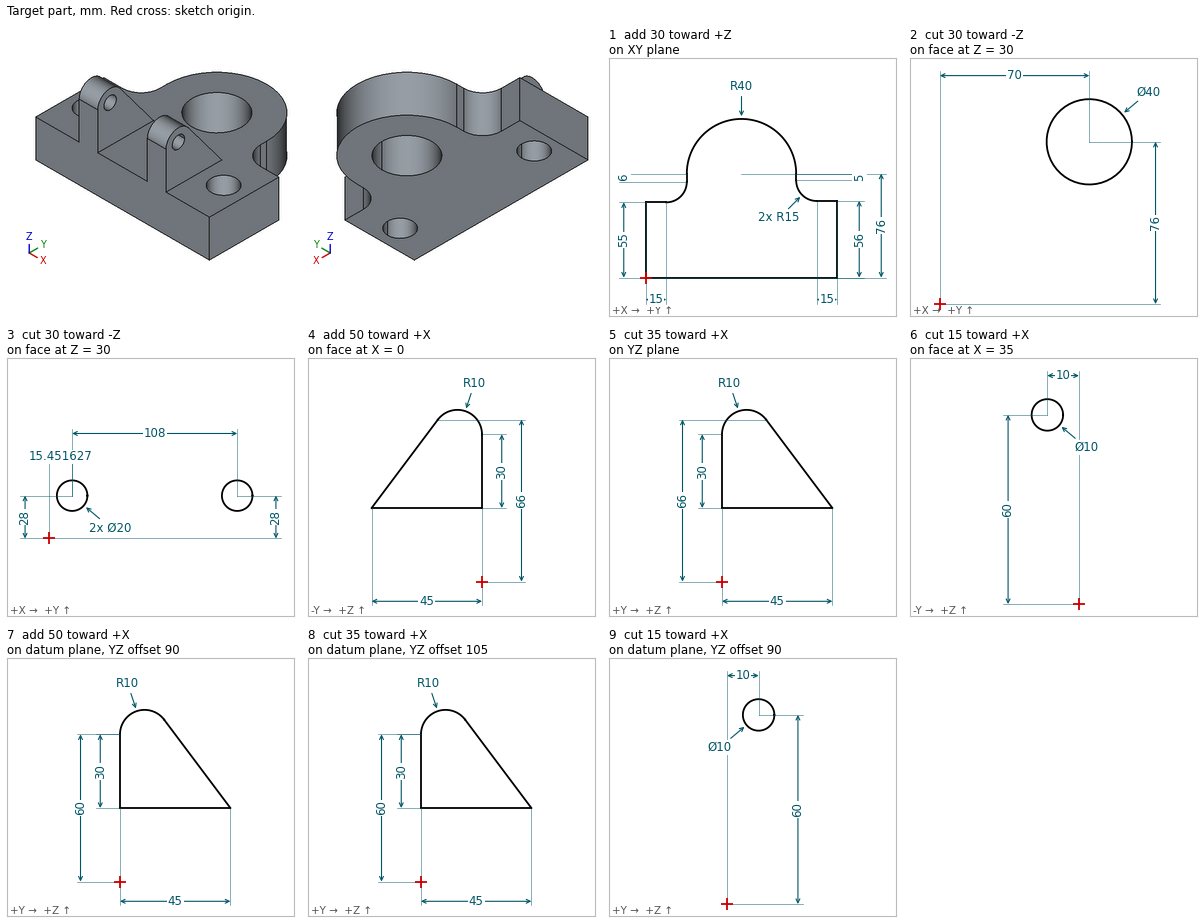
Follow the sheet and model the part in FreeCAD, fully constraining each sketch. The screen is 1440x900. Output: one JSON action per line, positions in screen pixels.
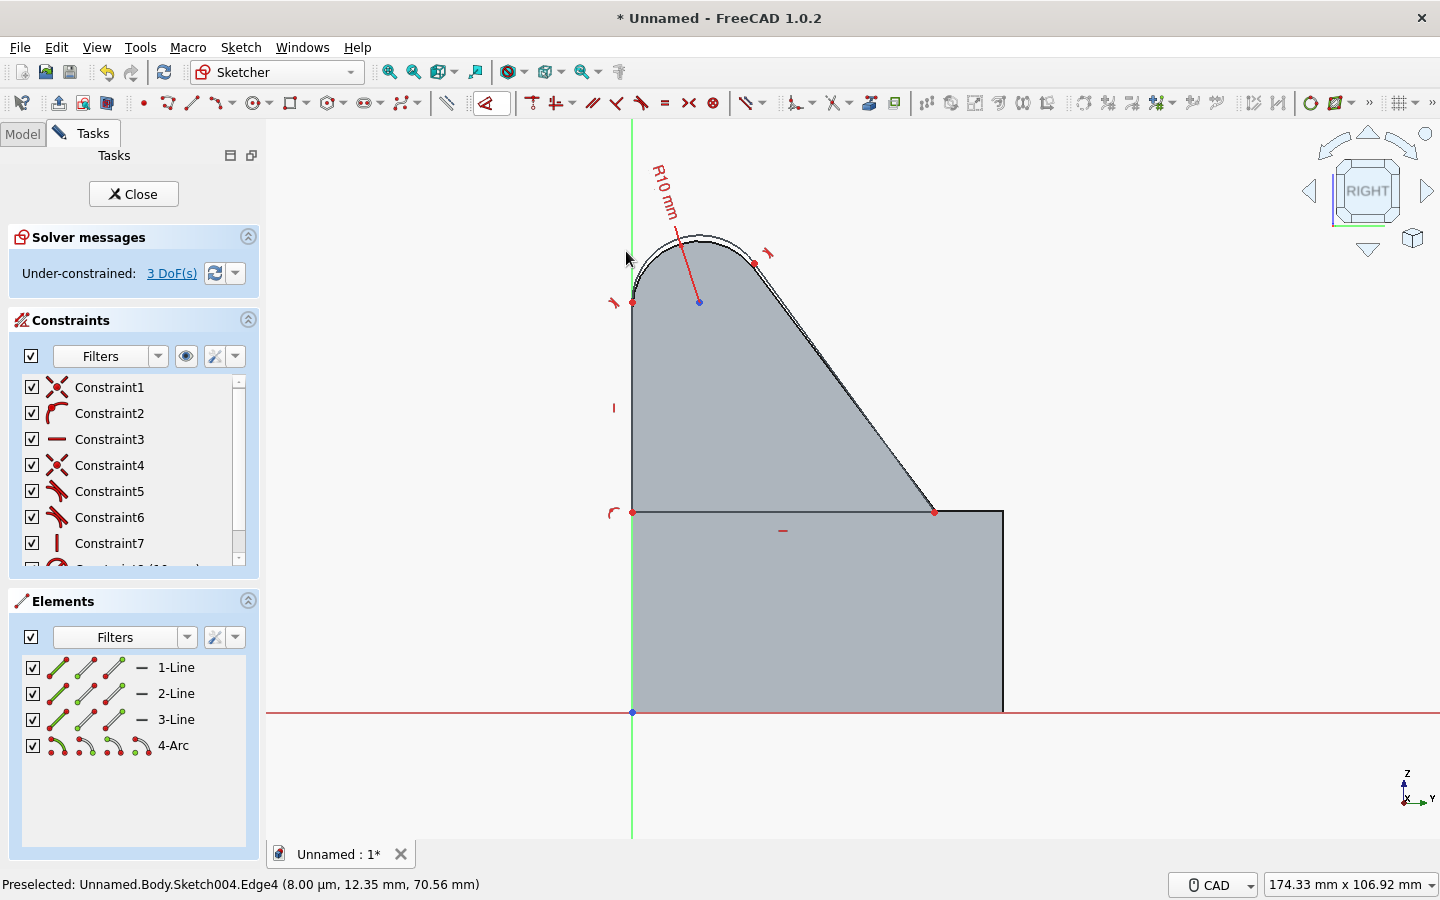
{"action": "left_click", "coordinate": [844, 512]}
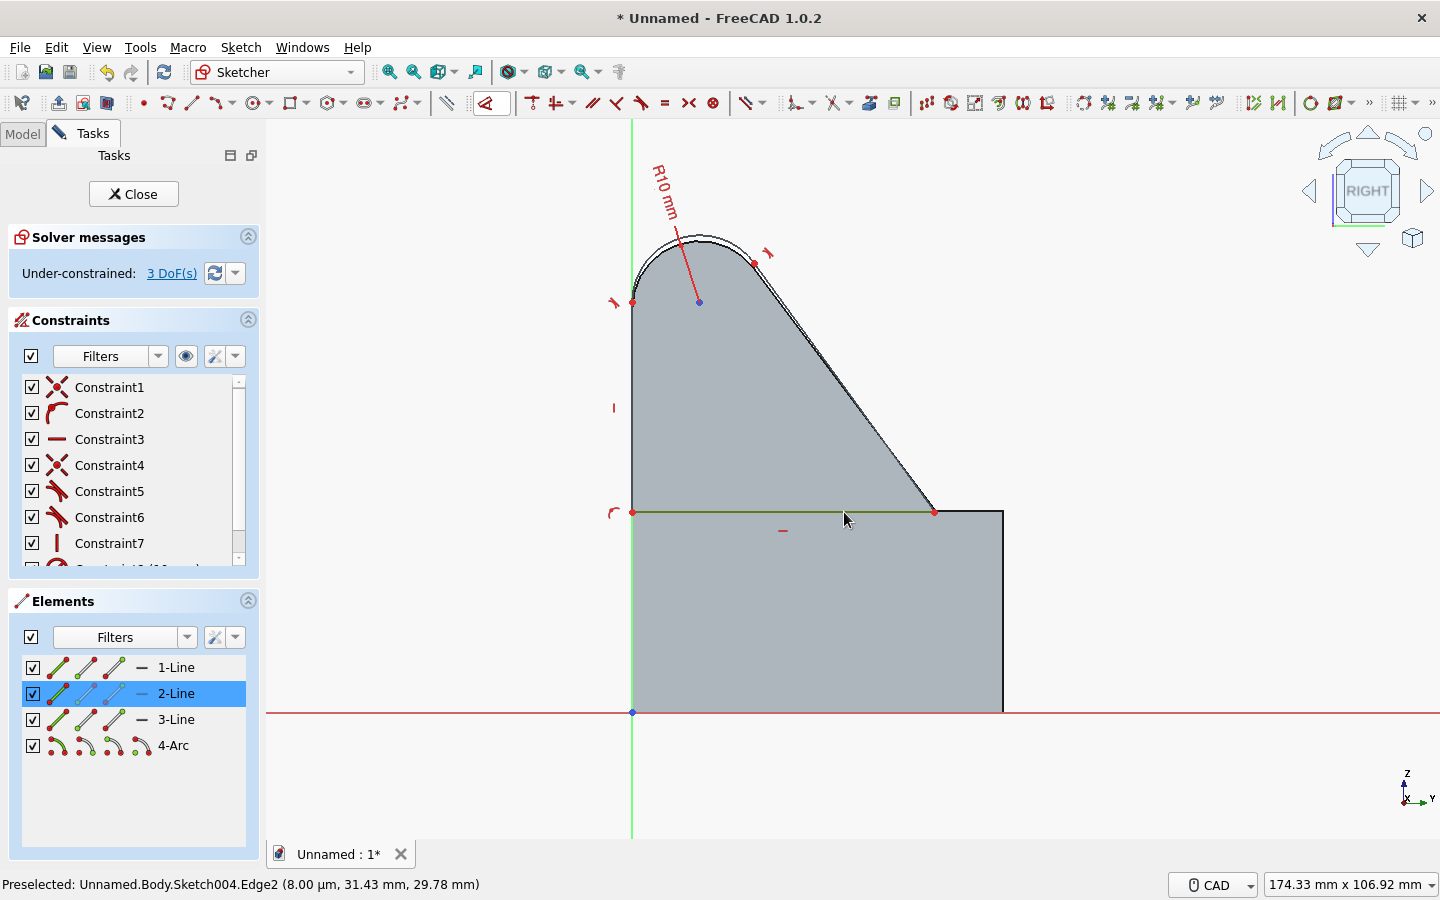
{"action": "left_click", "coordinate": [504, 104]}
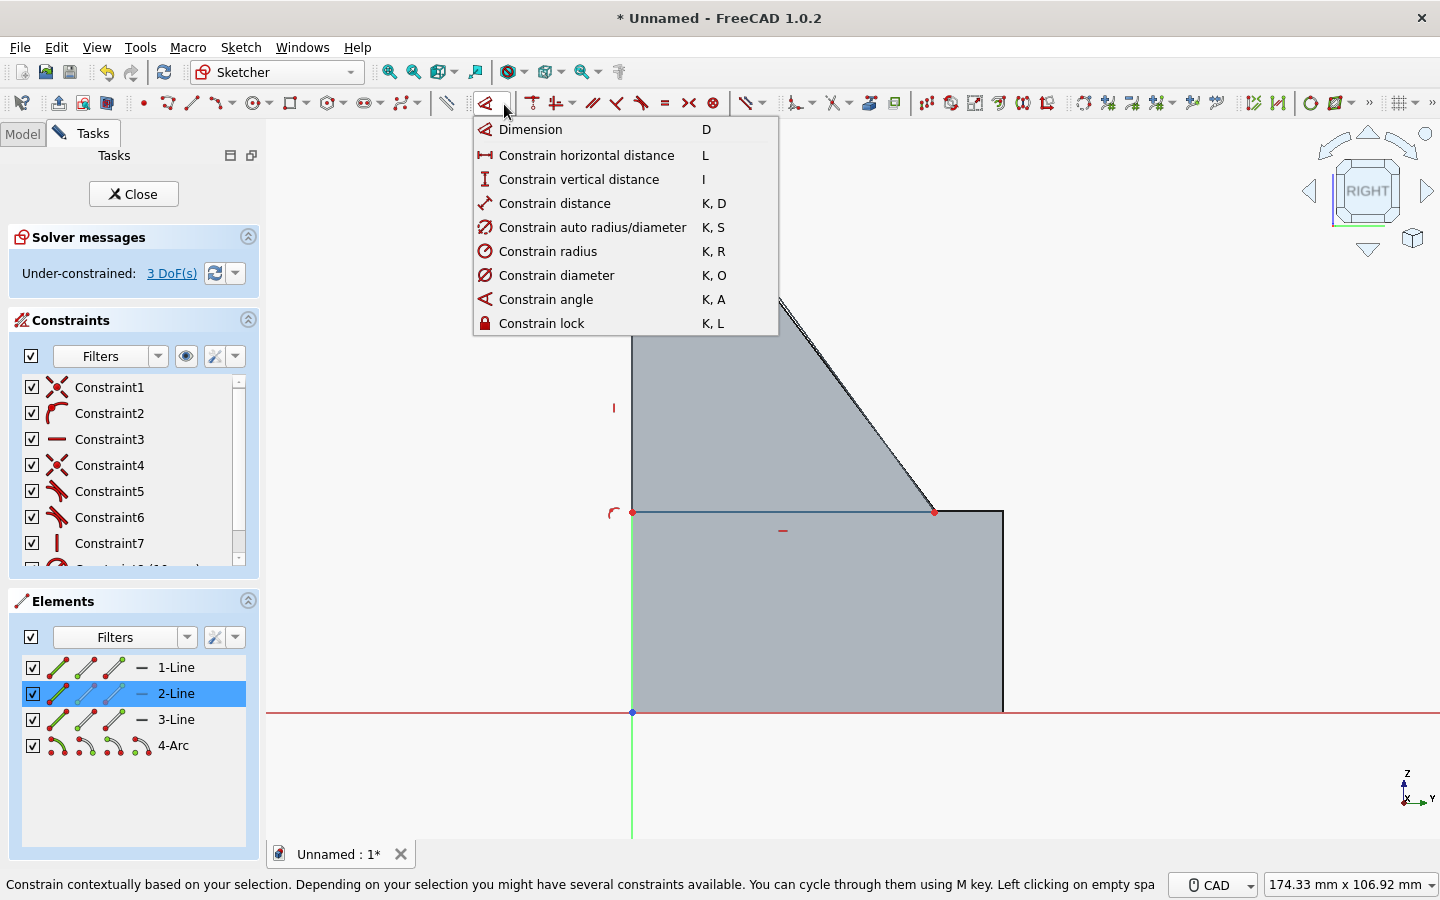
{"action": "left_click", "coordinate": [626, 155]}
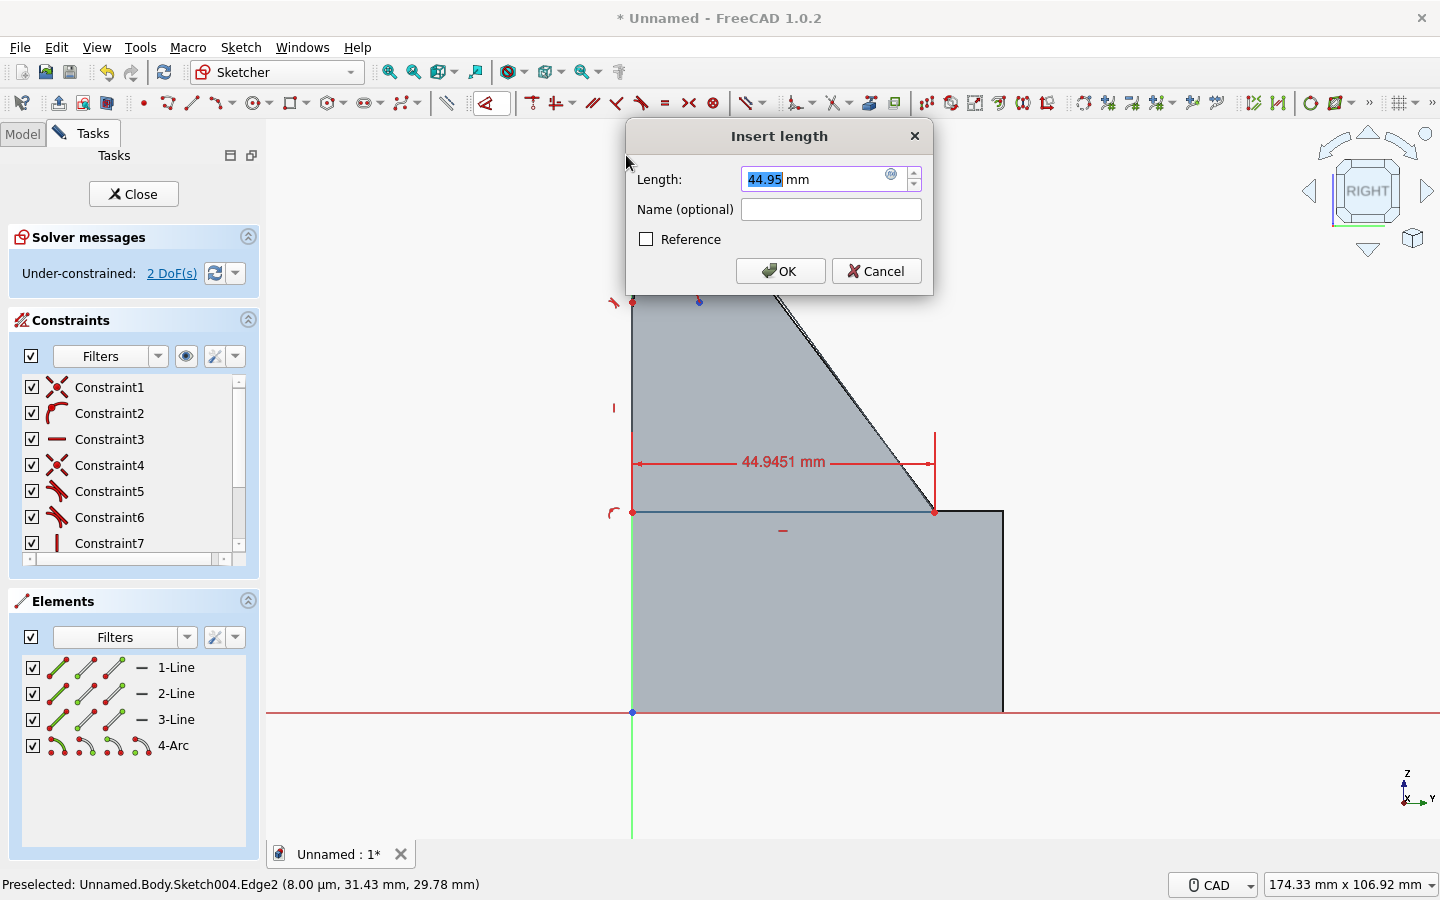
{"action": "type", "text": "45"}
{"action": "key", "text": "Return"}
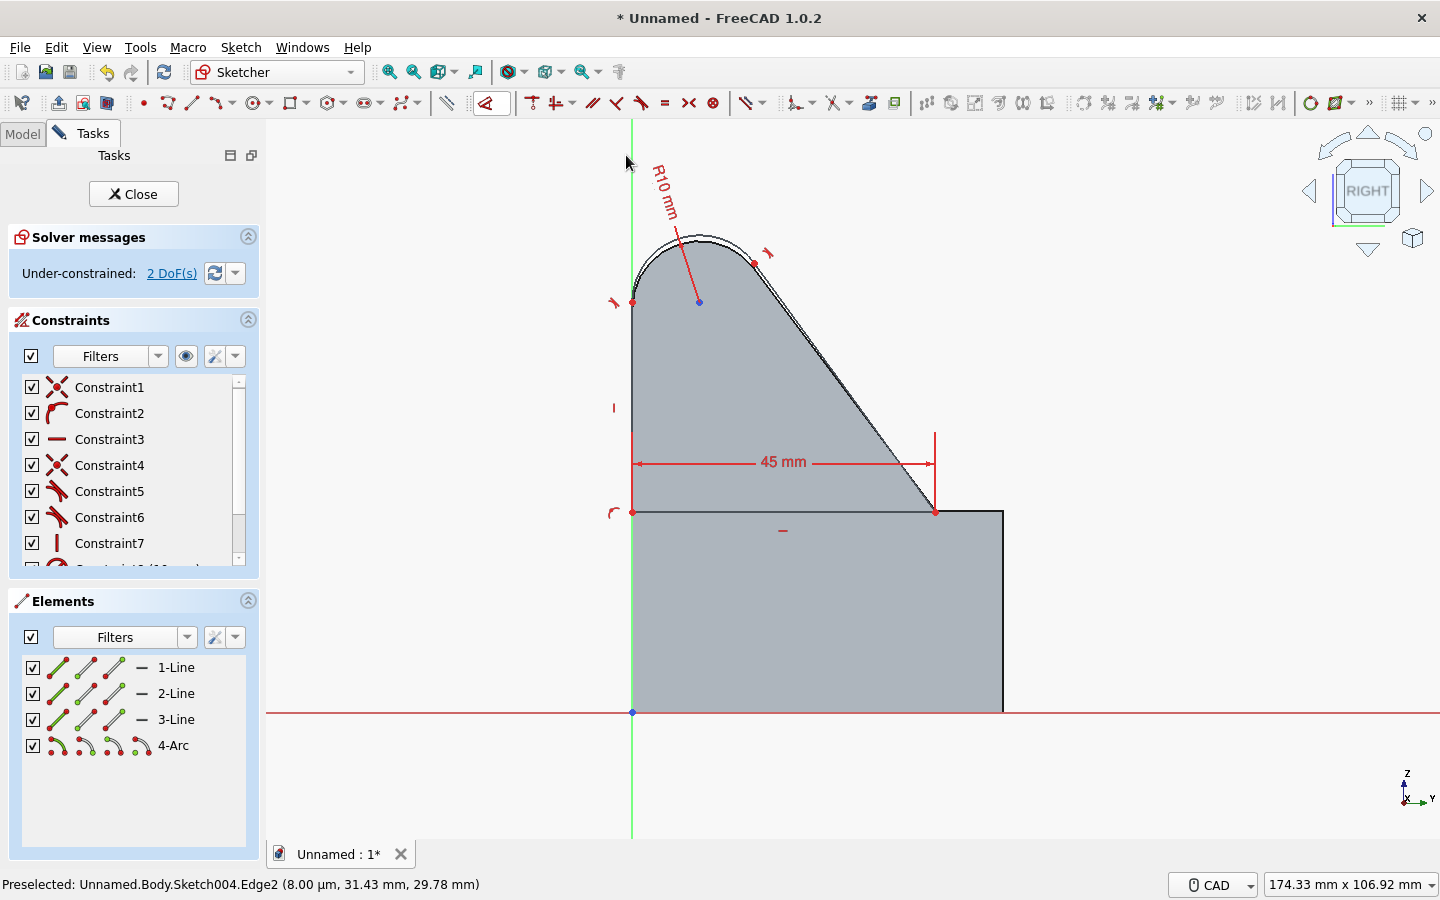
{"action": "left_click", "coordinate": [632, 449]}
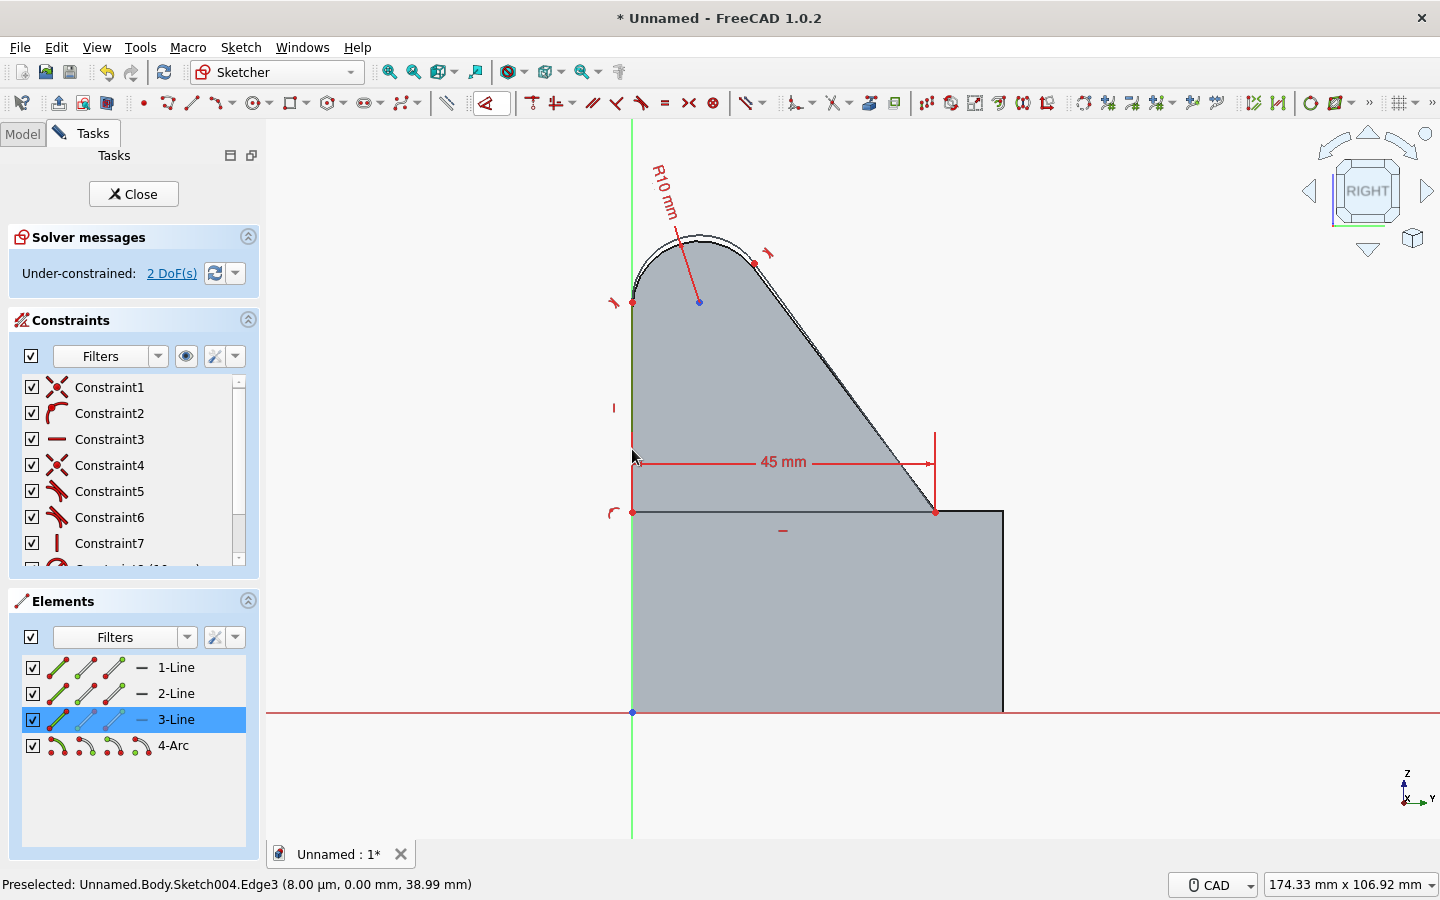
{"action": "left_click", "coordinate": [504, 104]}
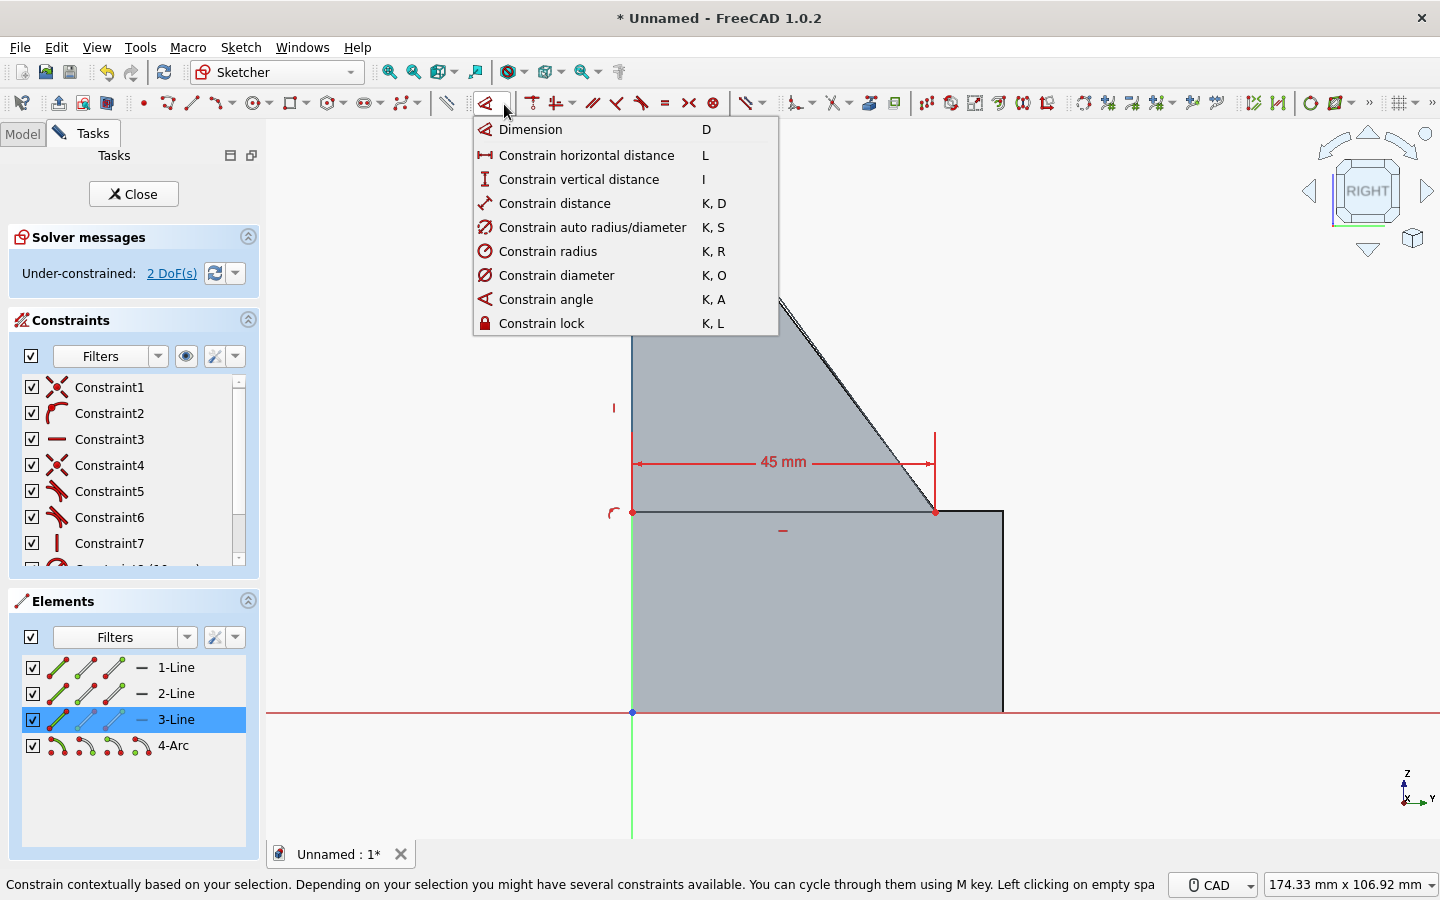
{"action": "left_click", "coordinate": [626, 179]}